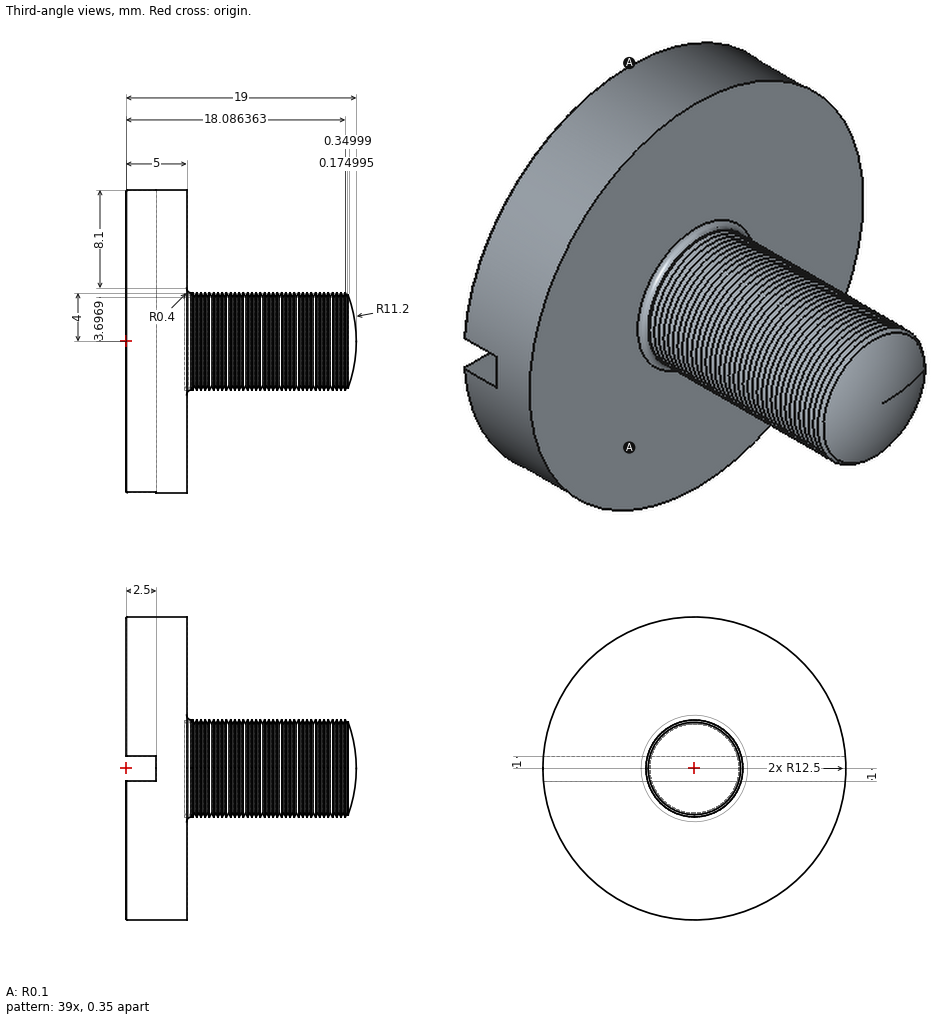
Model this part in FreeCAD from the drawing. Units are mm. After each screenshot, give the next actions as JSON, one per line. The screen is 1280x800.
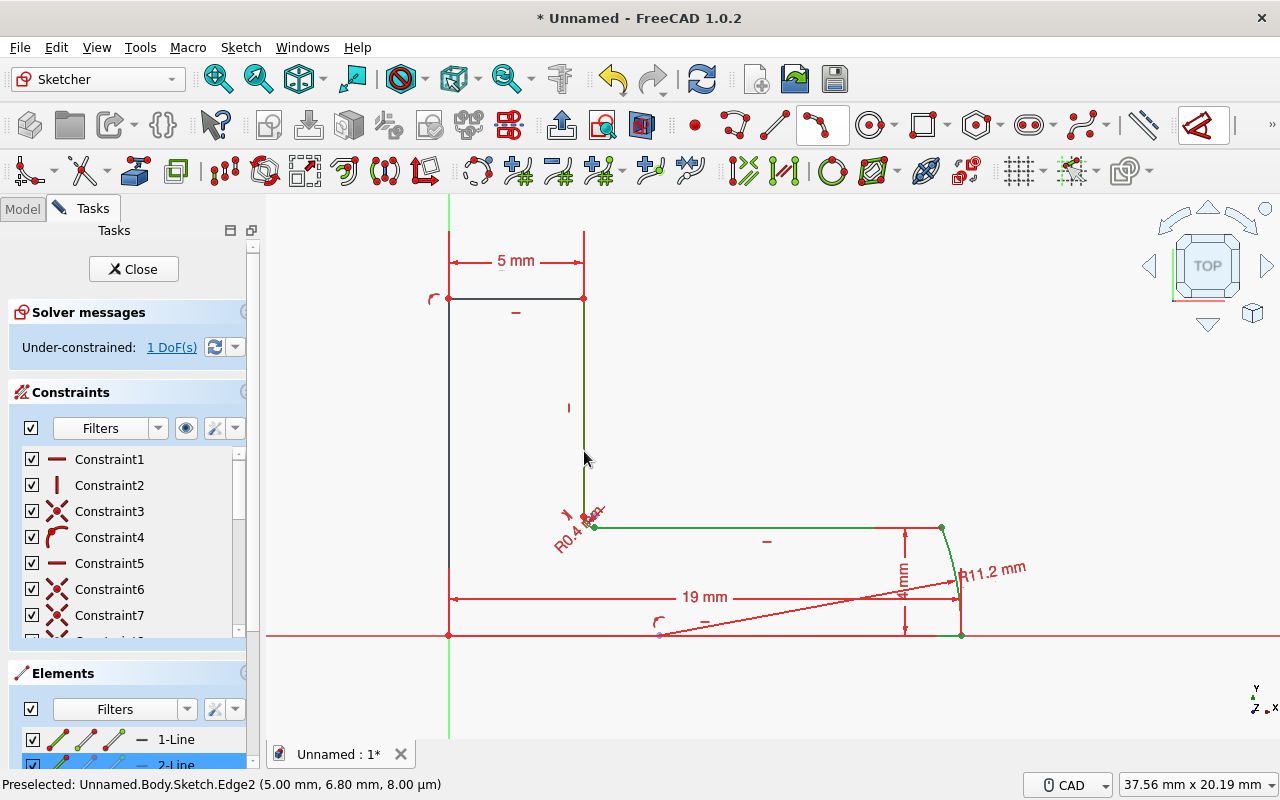
{"action": "key", "text": "i"}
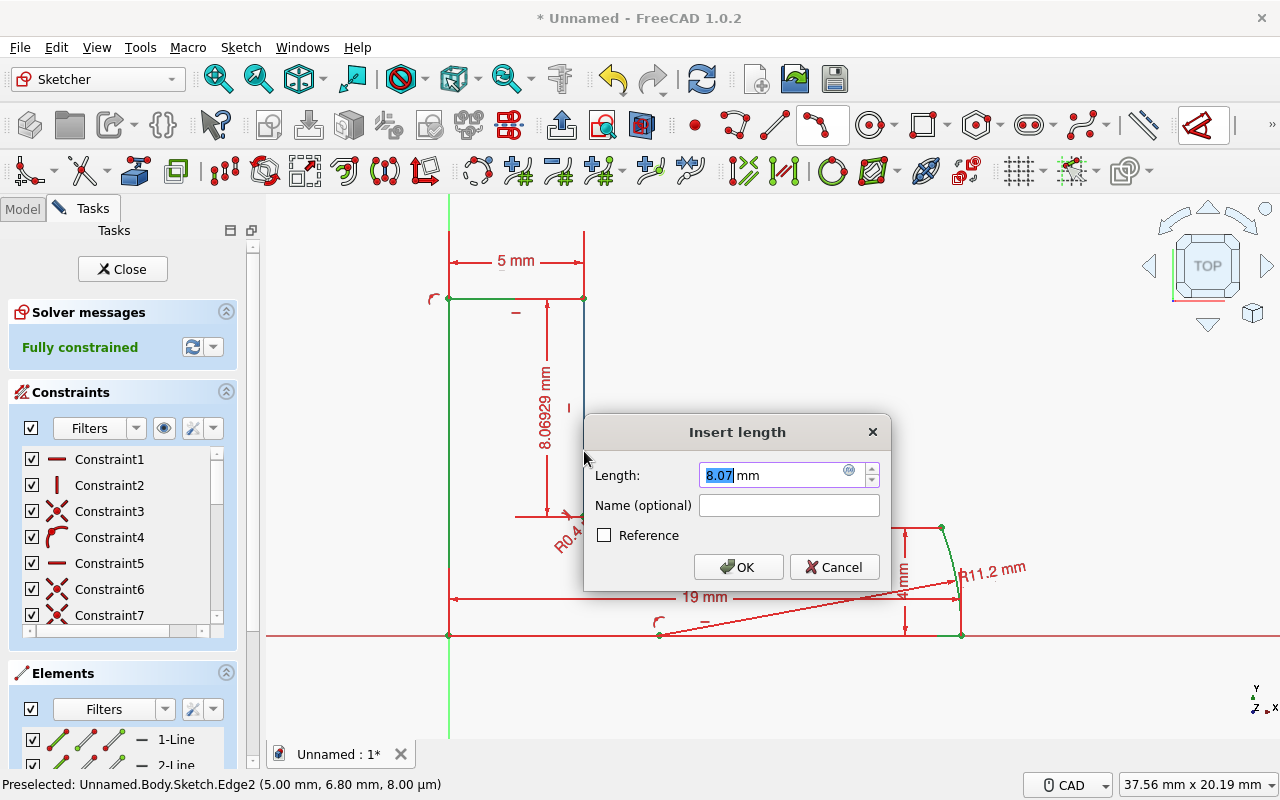
{"action": "type", "text": "8.1"}
{"action": "key", "text": "Return"}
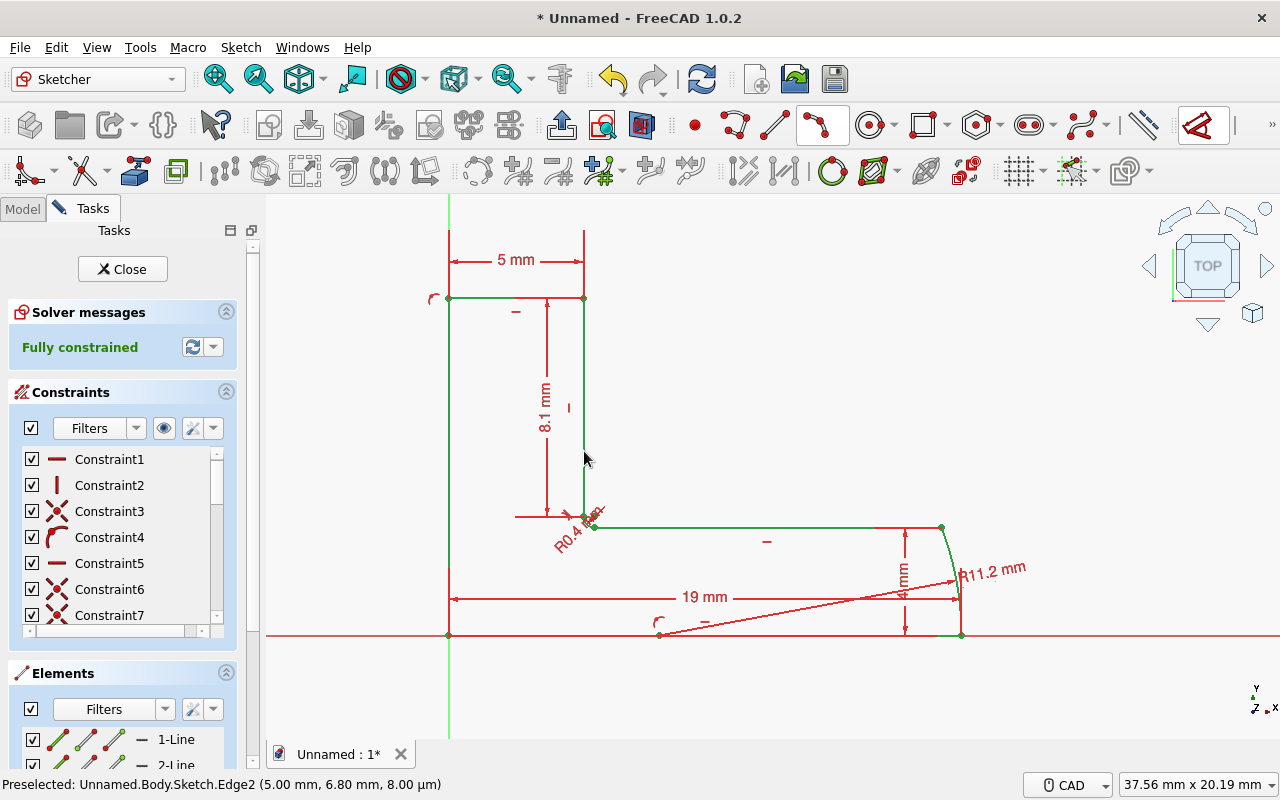
{"action": "left_click", "coordinate": [123, 269]}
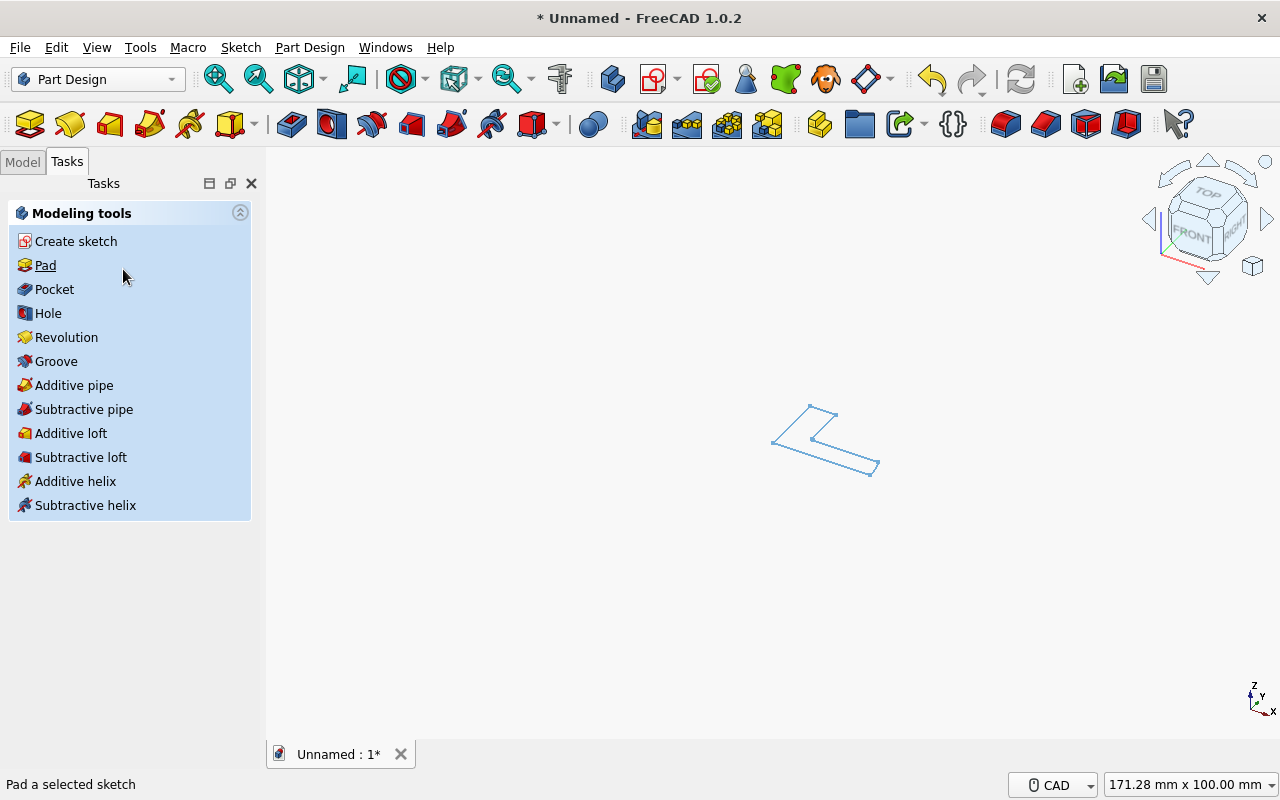
{"action": "left_click", "coordinate": [70, 124]}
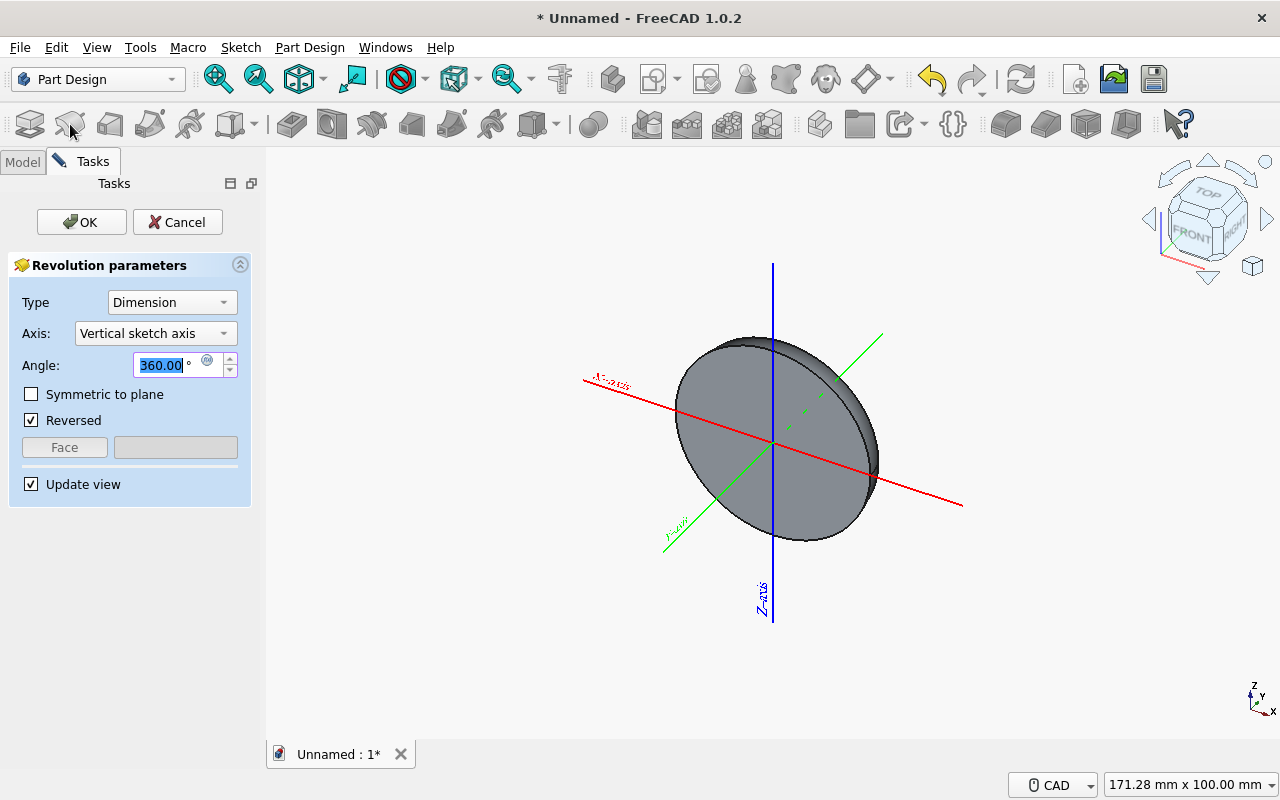
{"action": "left_click", "coordinate": [156, 334]}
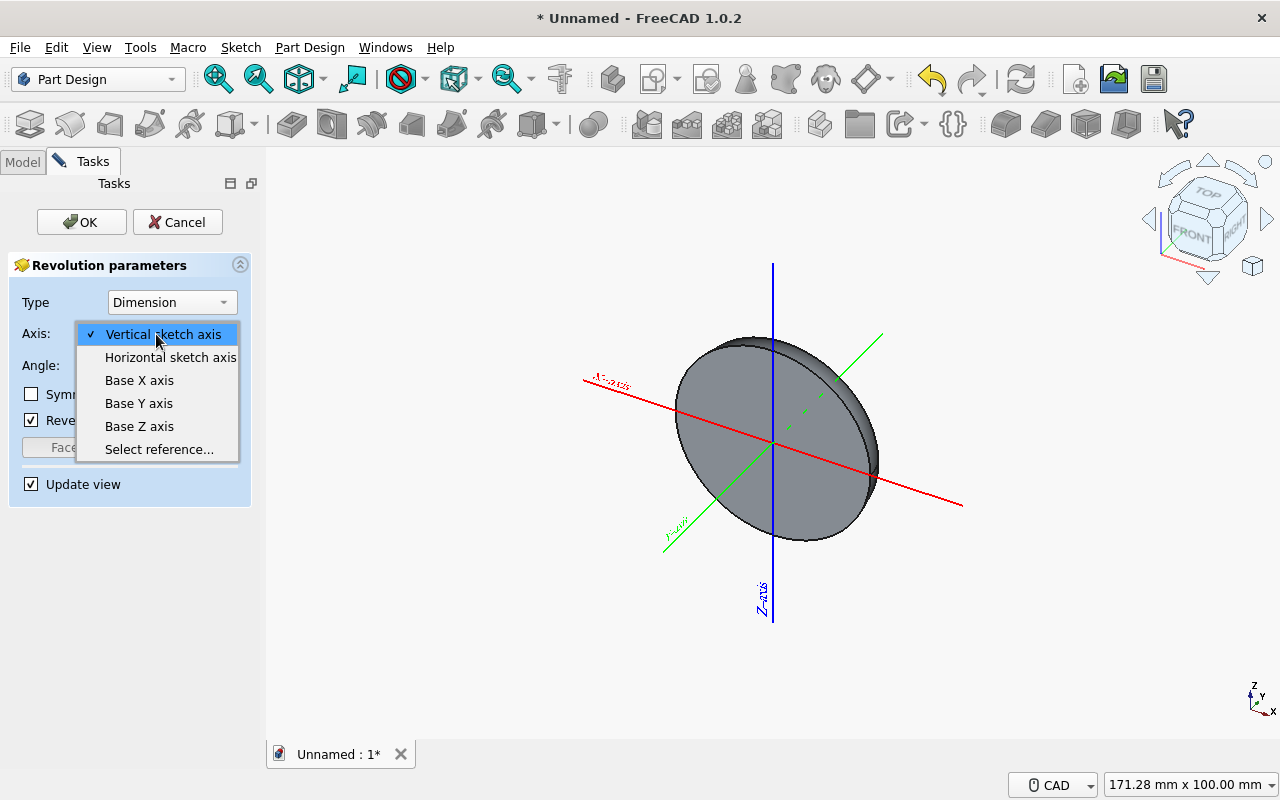
{"action": "left_click", "coordinate": [156, 358]}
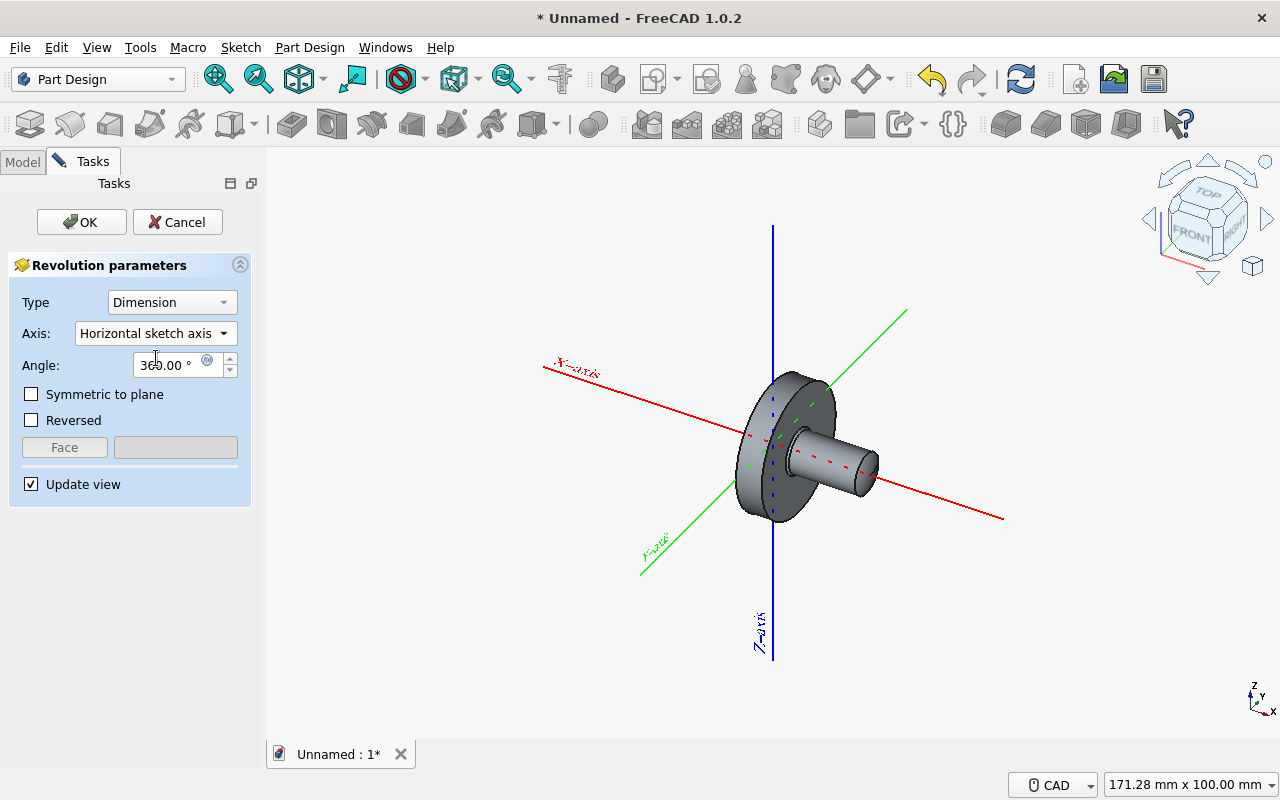
{"action": "left_click", "coordinate": [82, 222]}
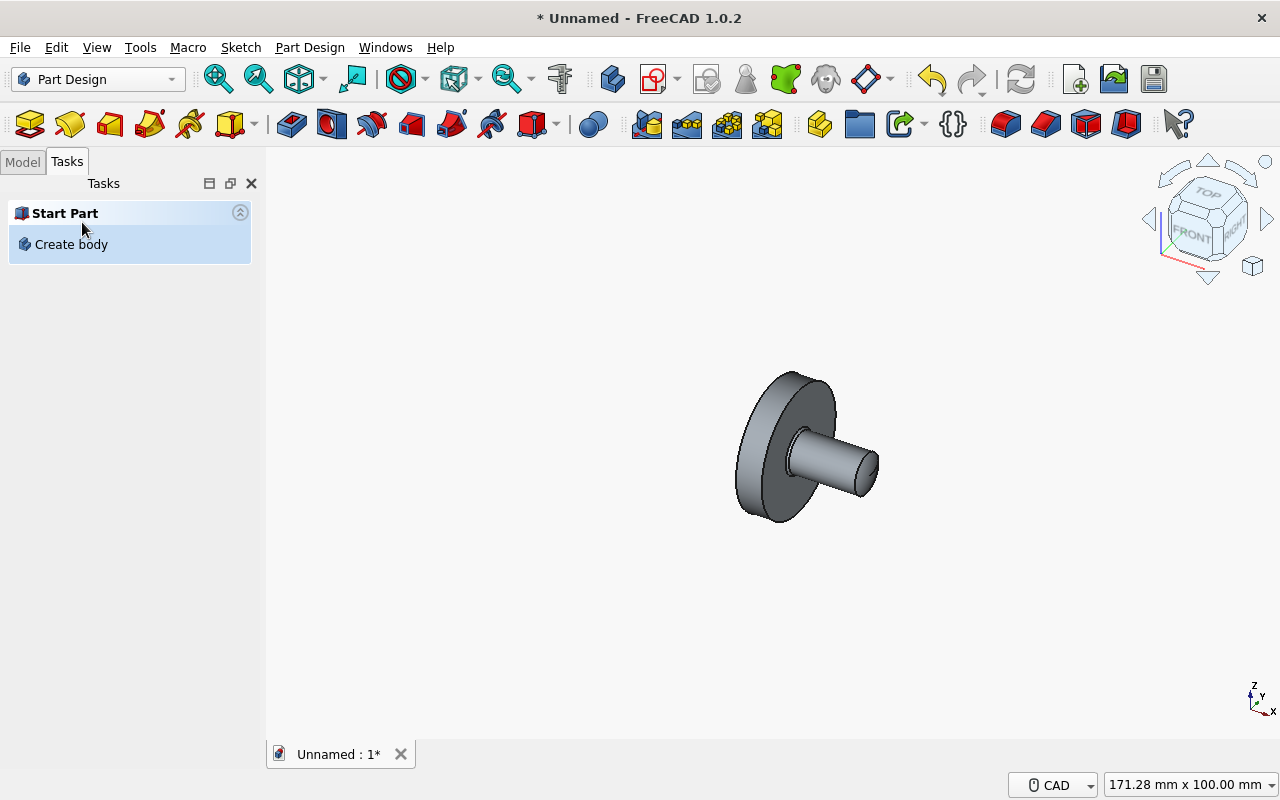
{"action": "left_click", "coordinate": [220, 80]}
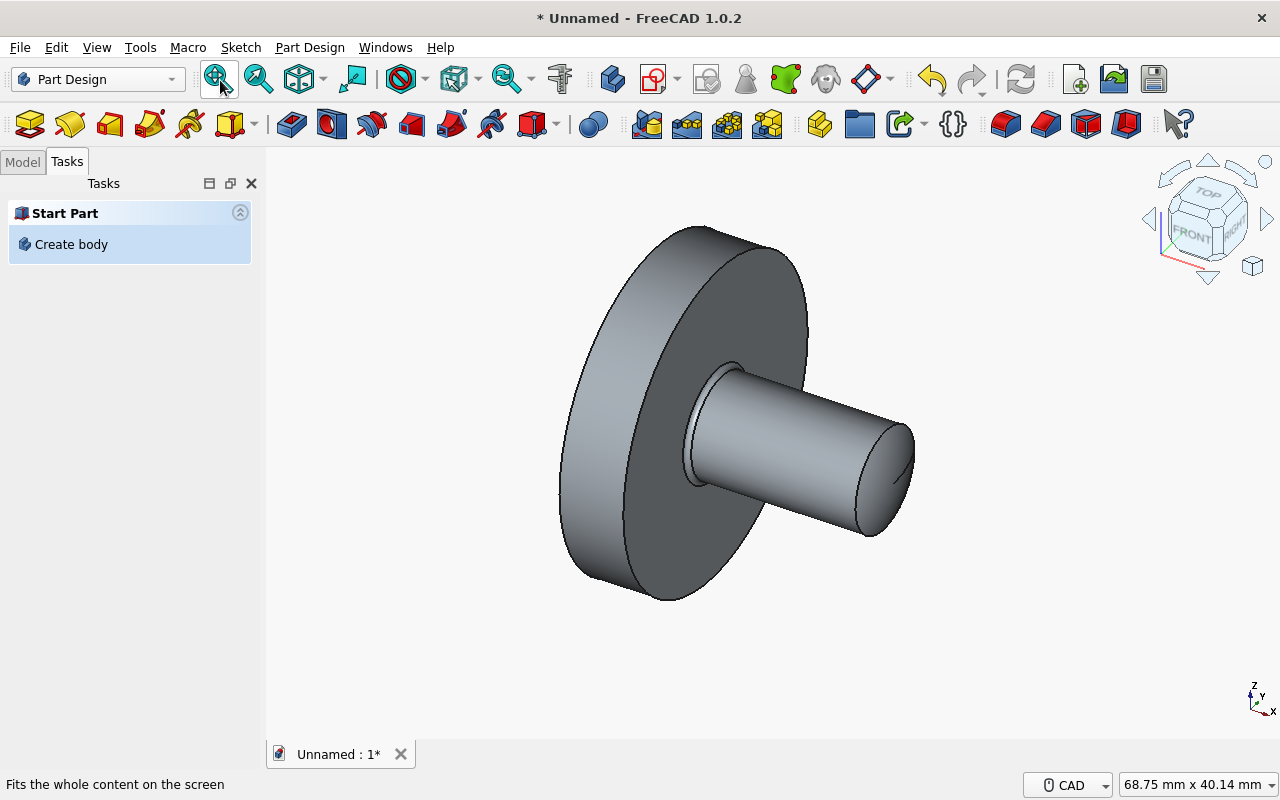
{"action": "left_click", "coordinate": [23, 161]}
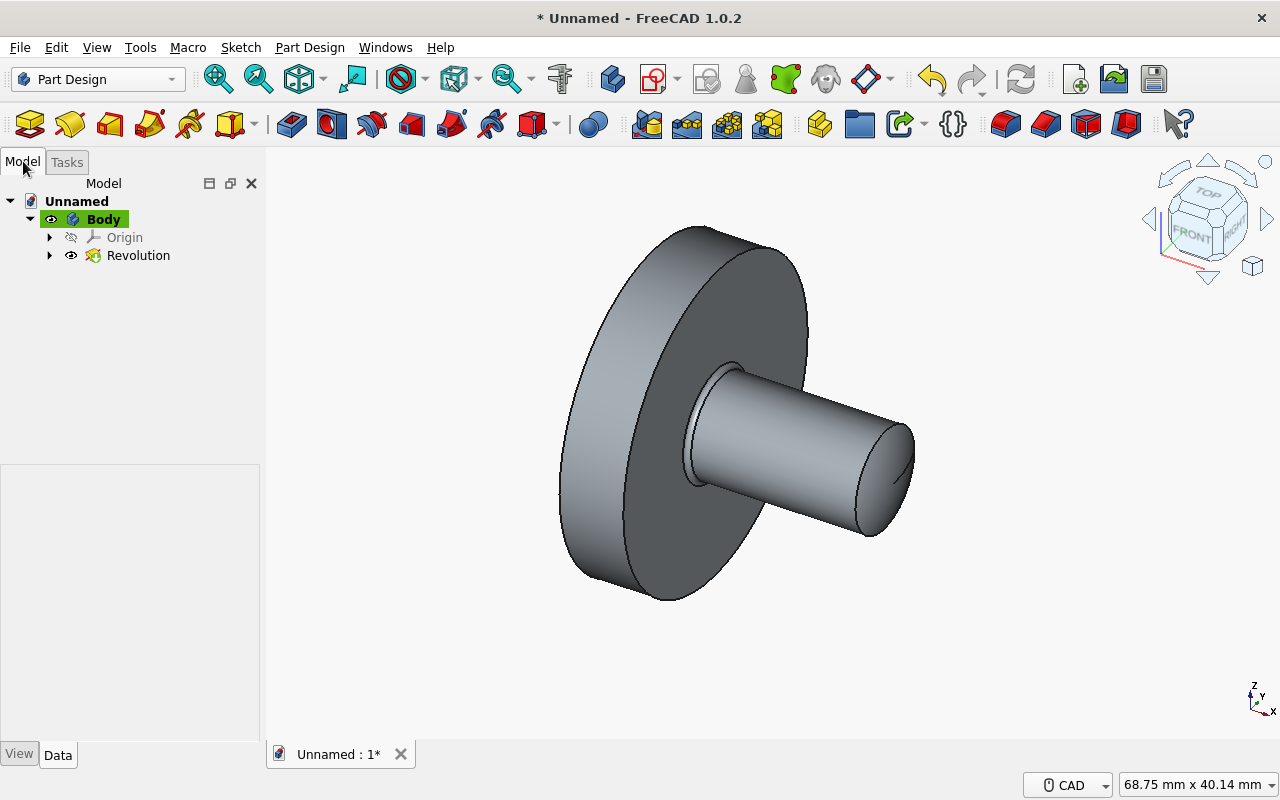
{"action": "left_click", "coordinate": [50, 237]}